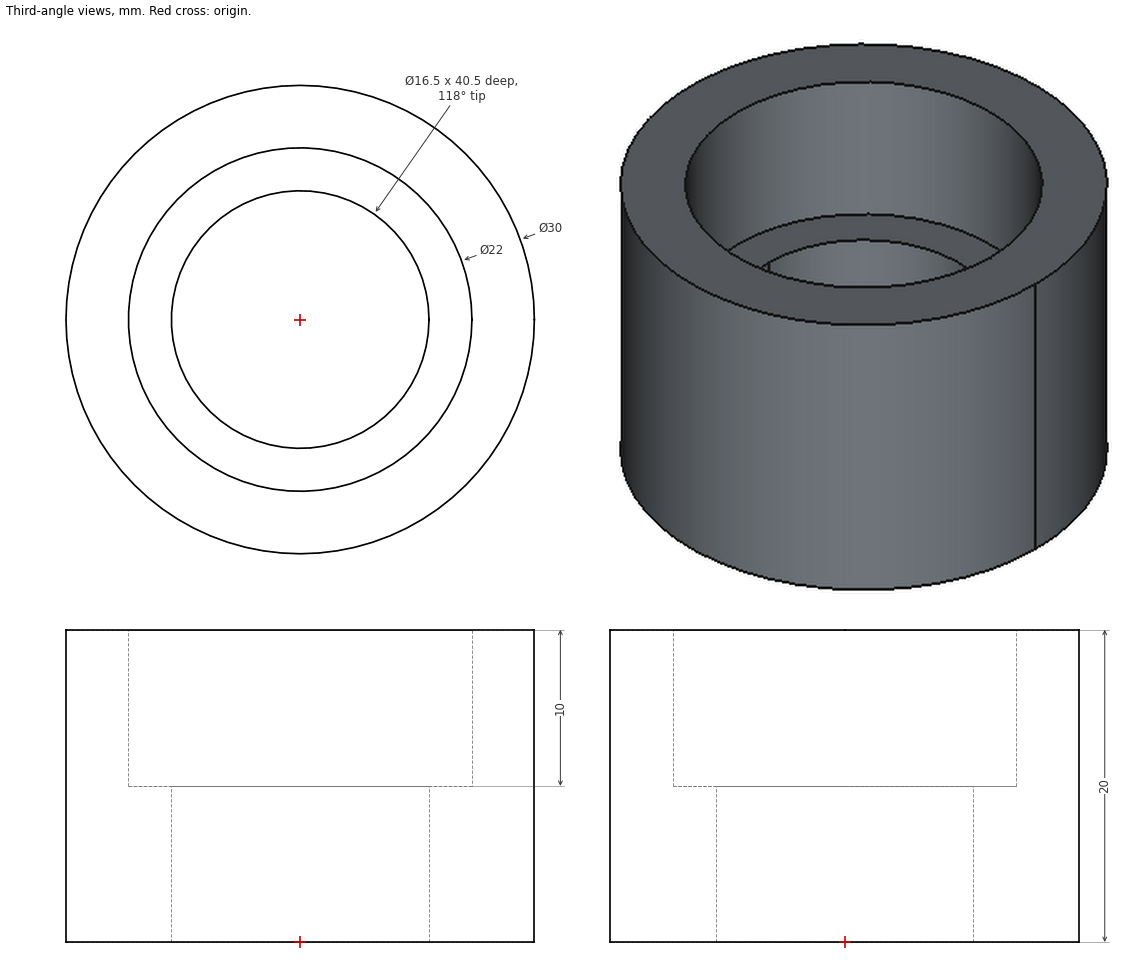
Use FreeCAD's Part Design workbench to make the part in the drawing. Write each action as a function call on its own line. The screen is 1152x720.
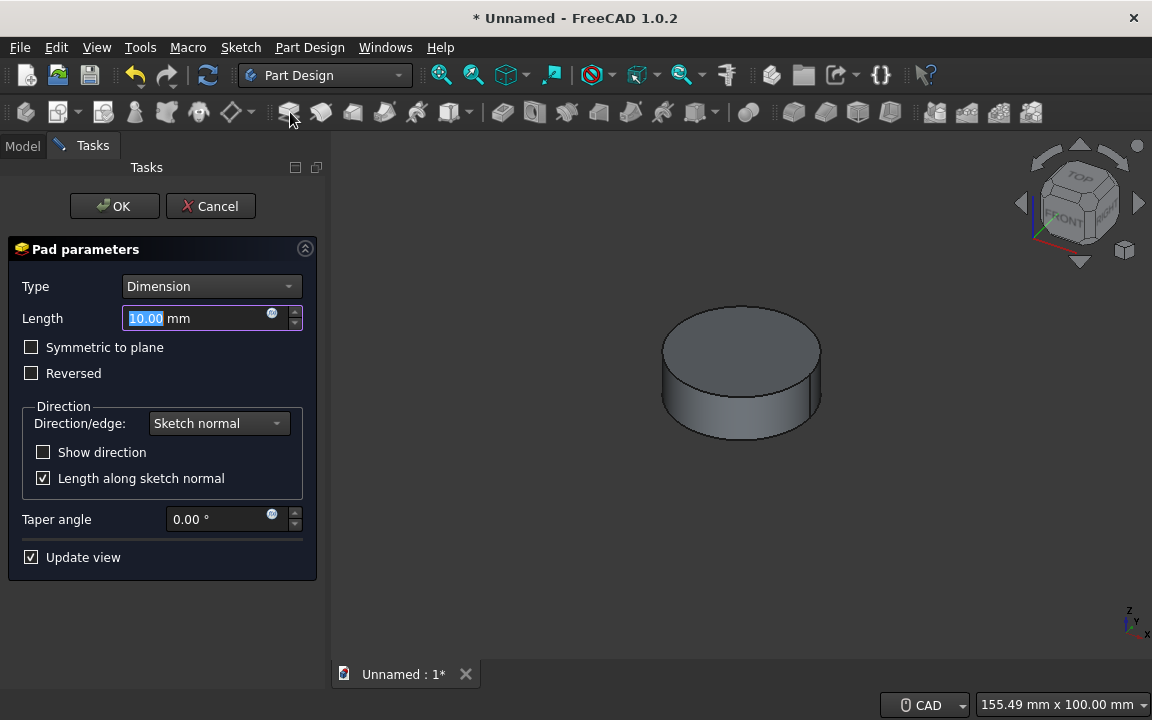
text(20)
key(Tab)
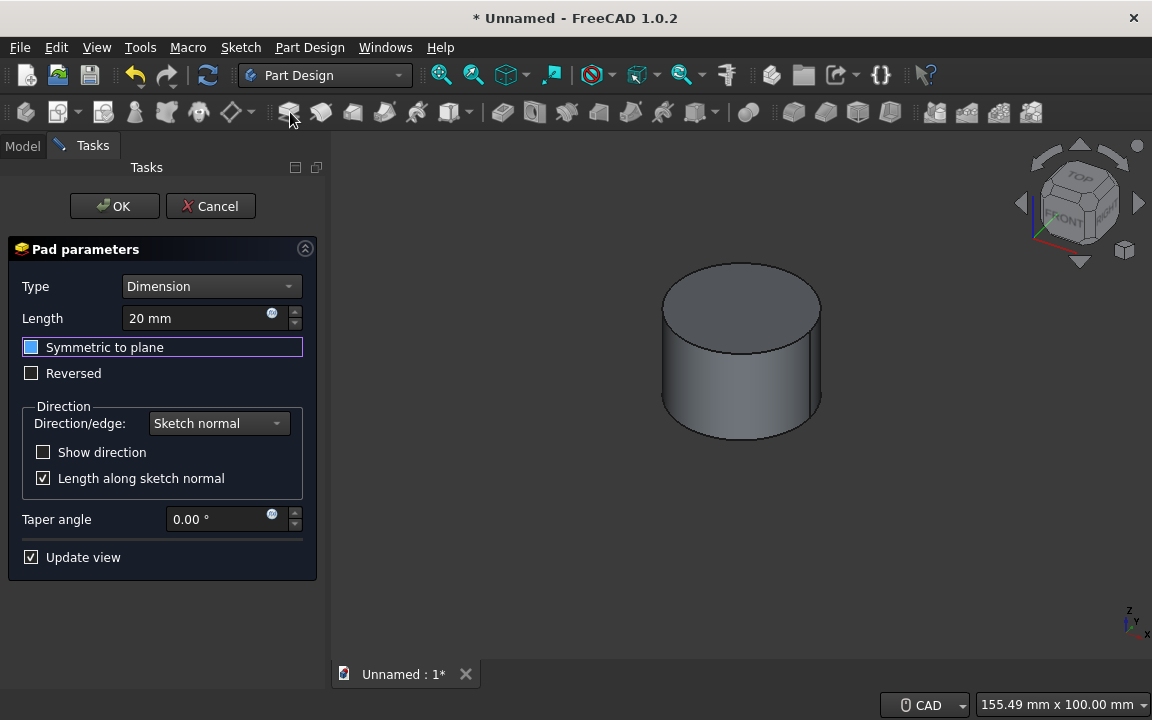
click(115, 206)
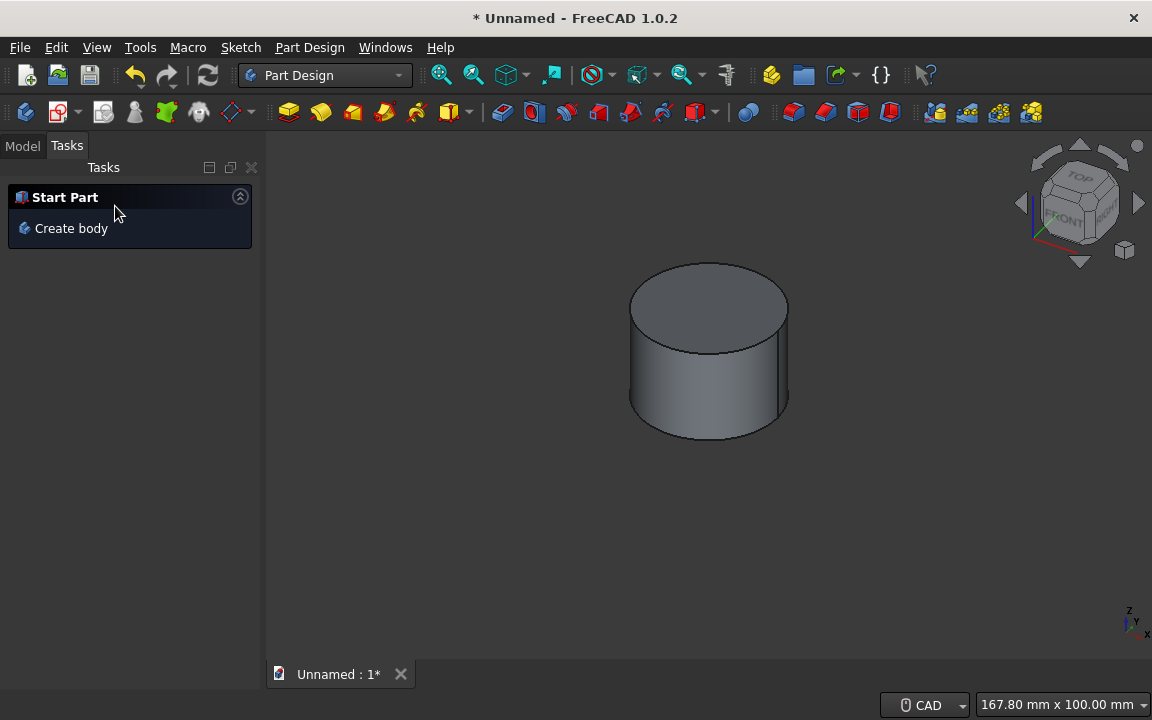
click(442, 76)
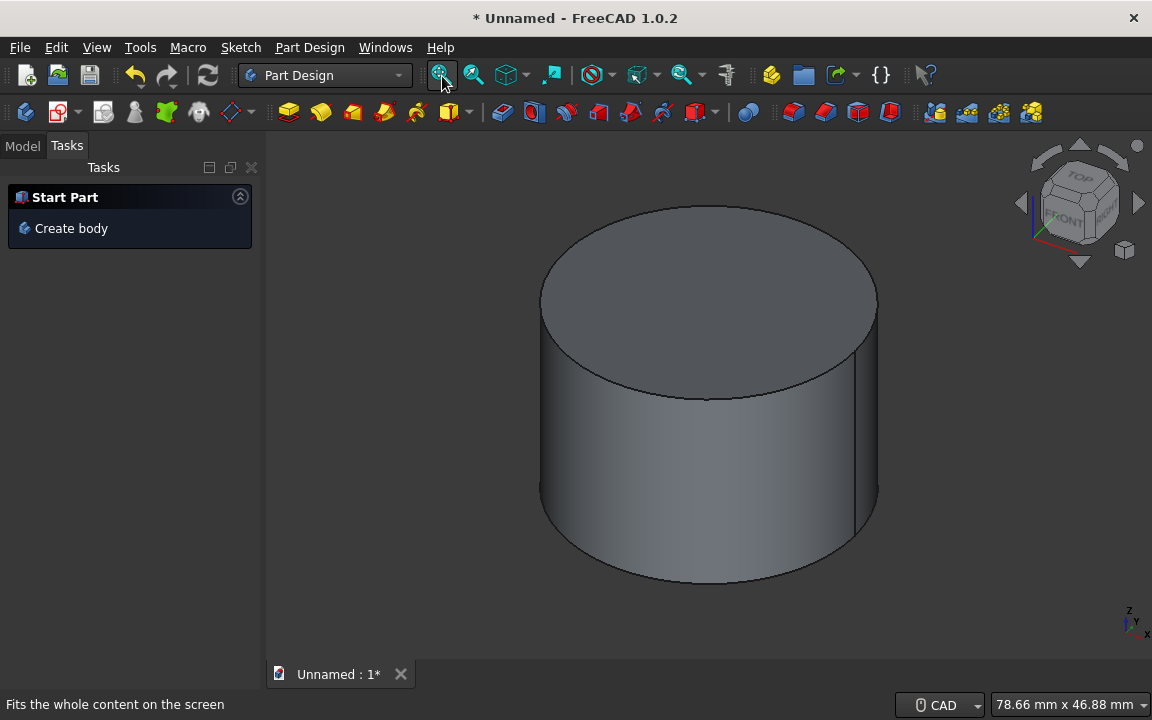
click(709, 302)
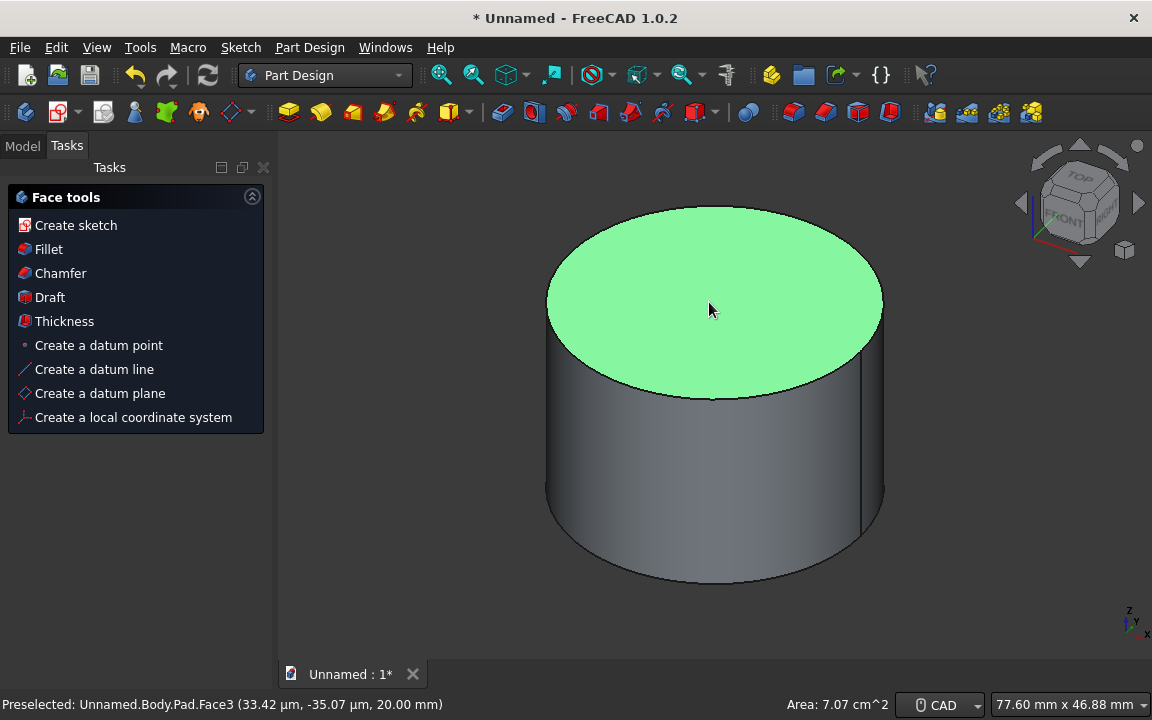
click(58, 112)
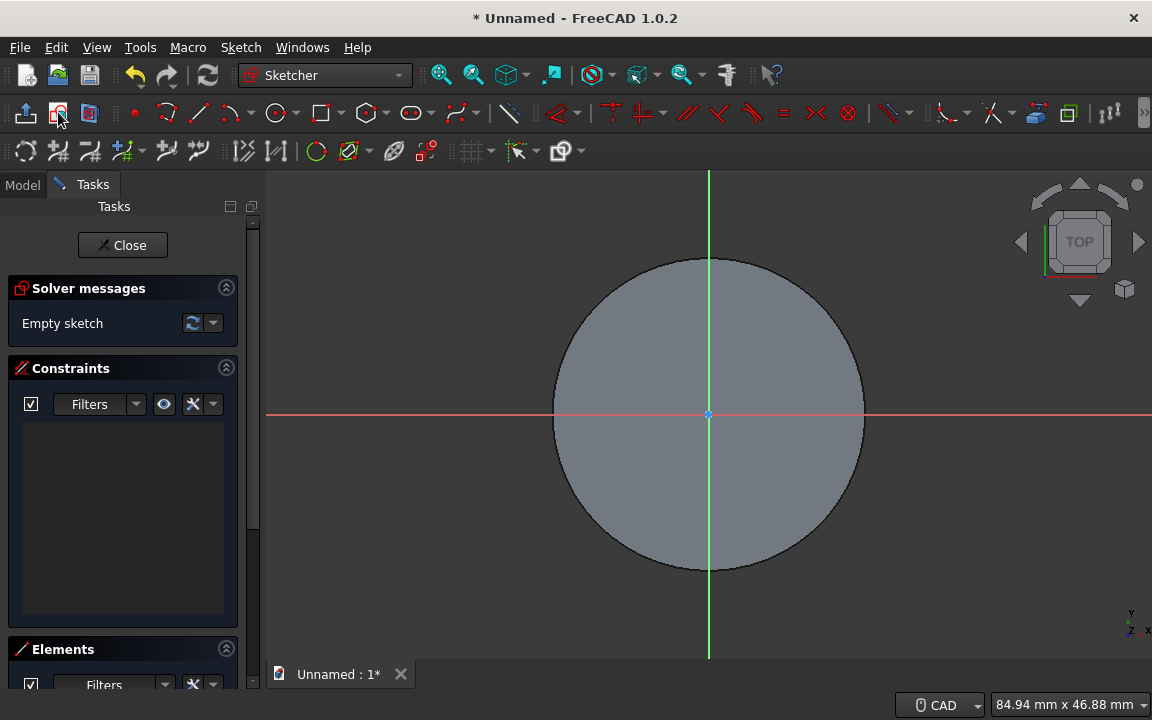
click(276, 114)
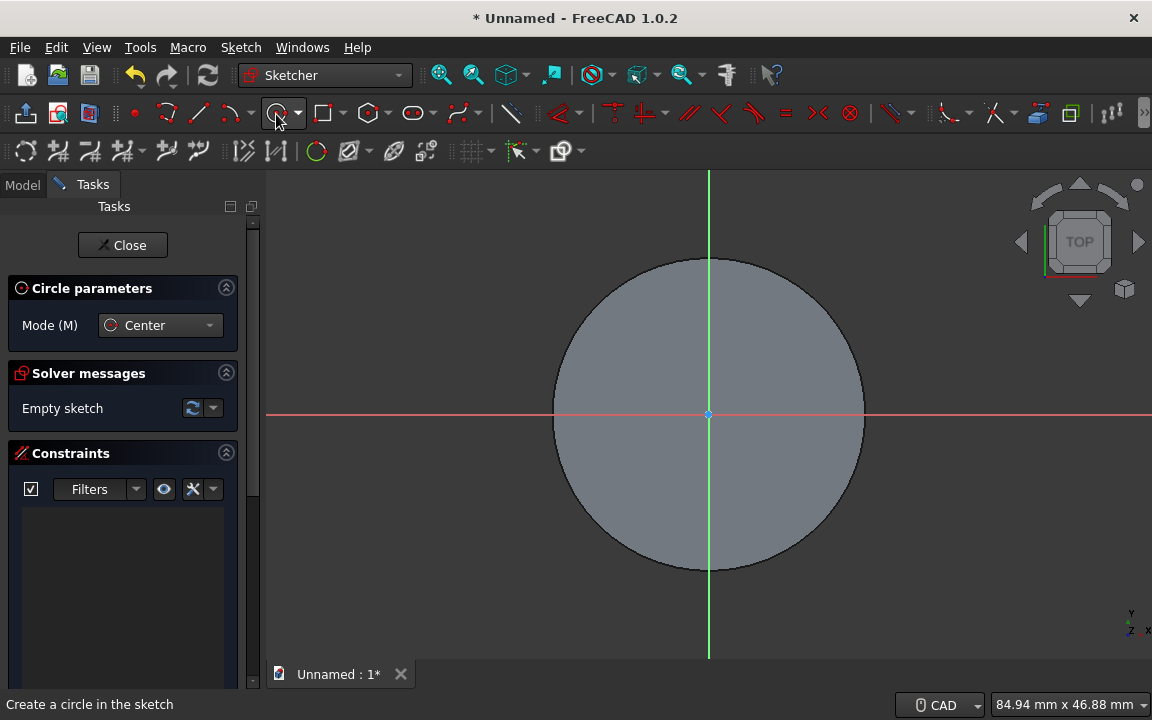
click(709, 414)
click(790, 333)
key(Escape)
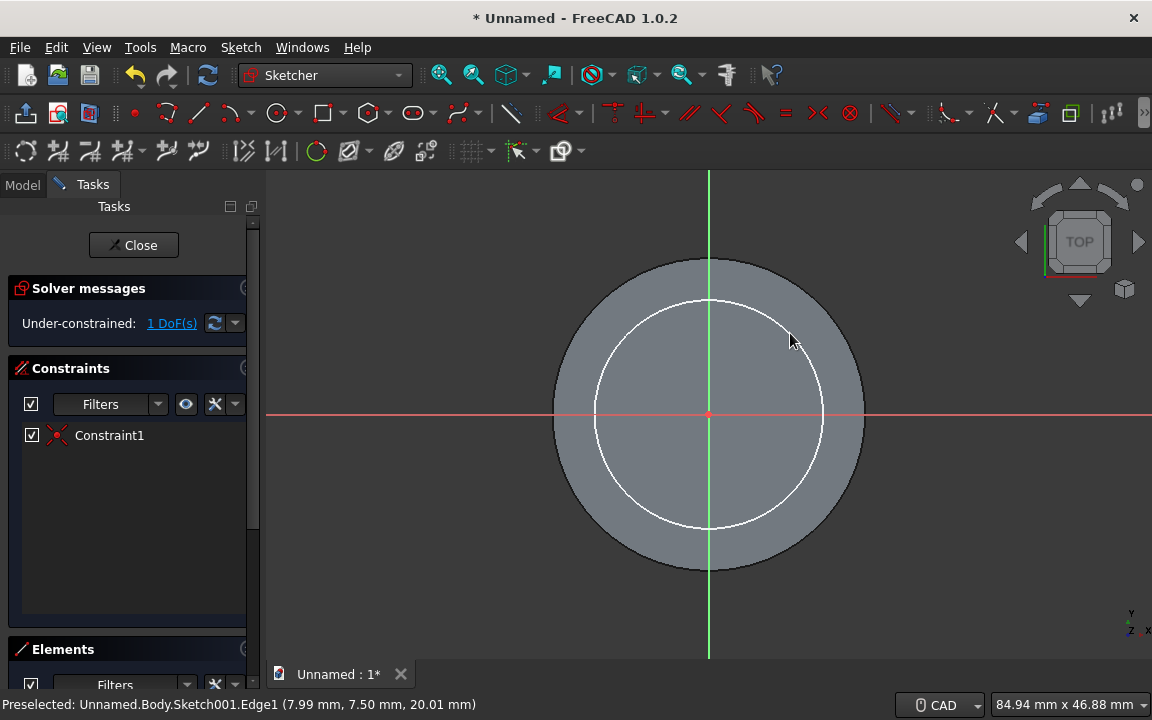
click(558, 114)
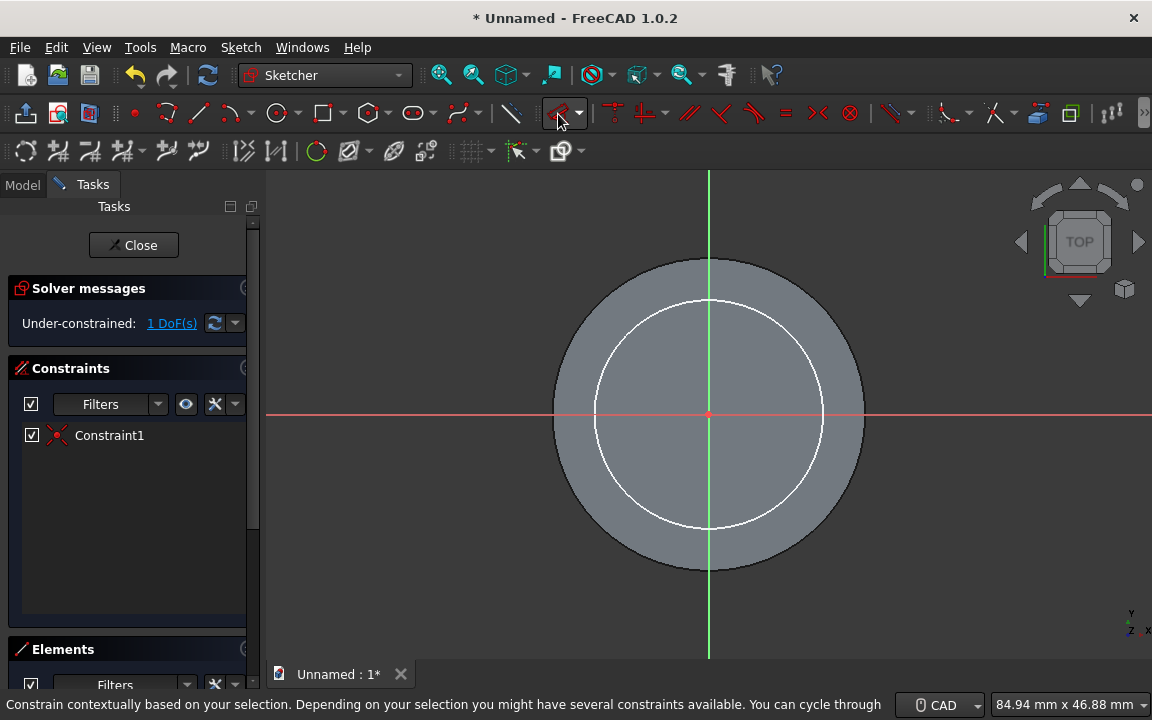
click(789, 333)
click(811, 310)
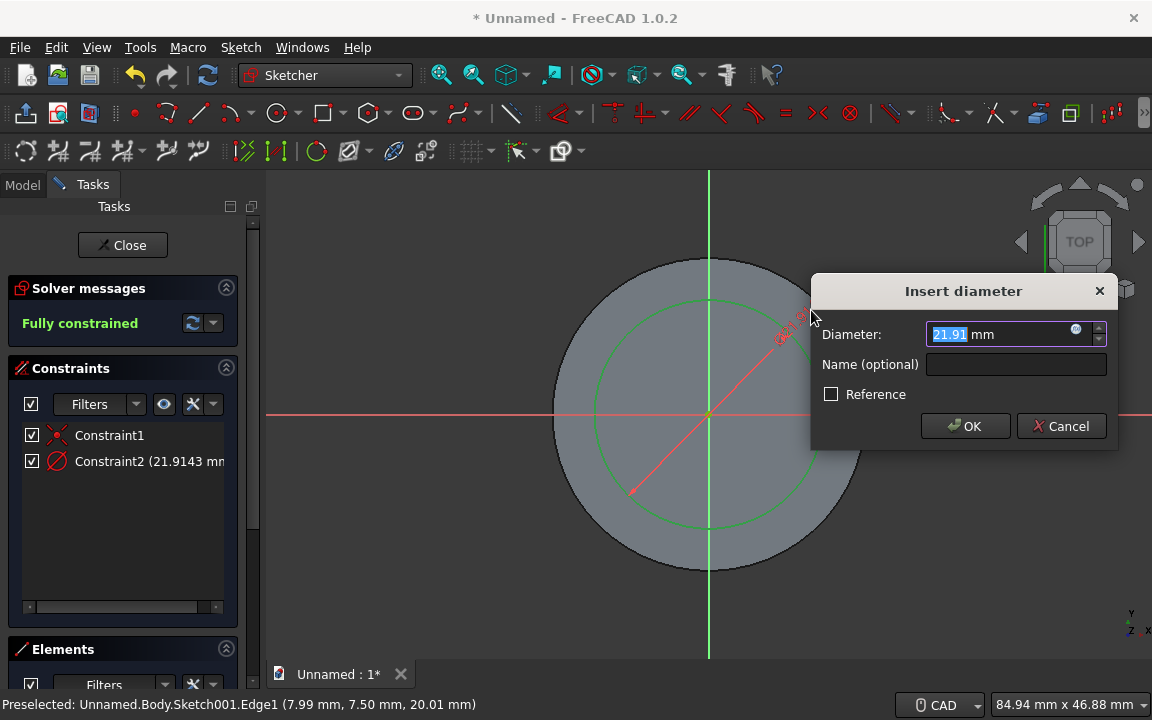
text(22)
key(Return)
key(Escape)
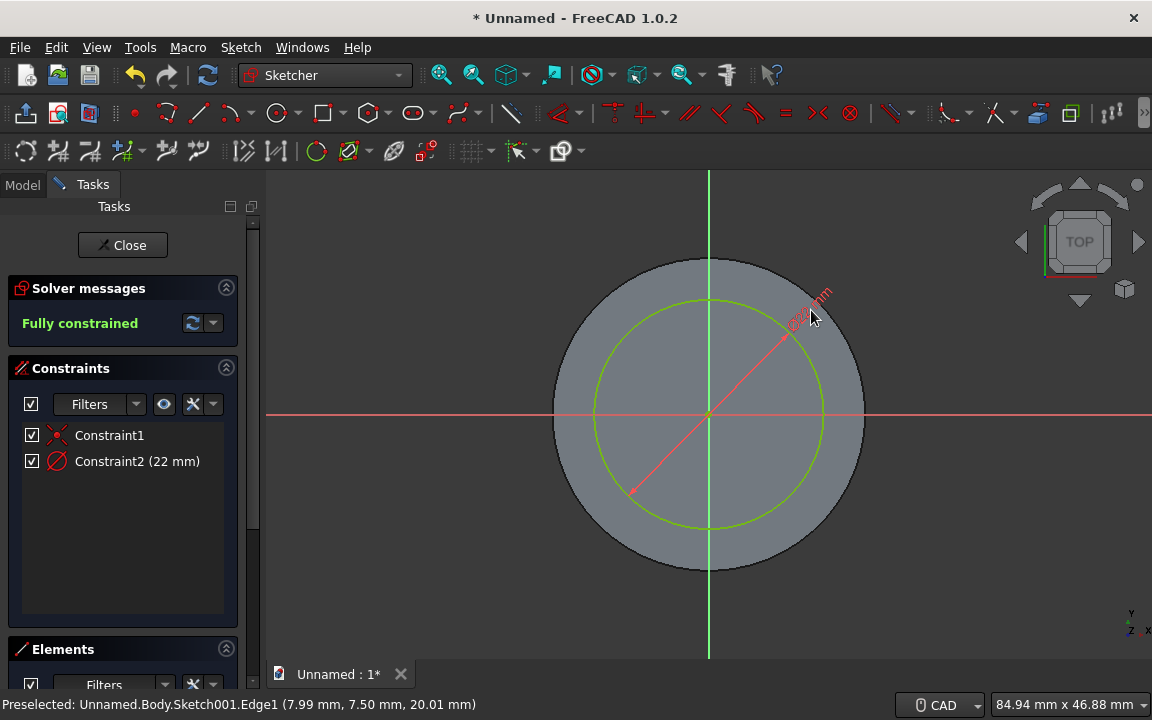
click(123, 245)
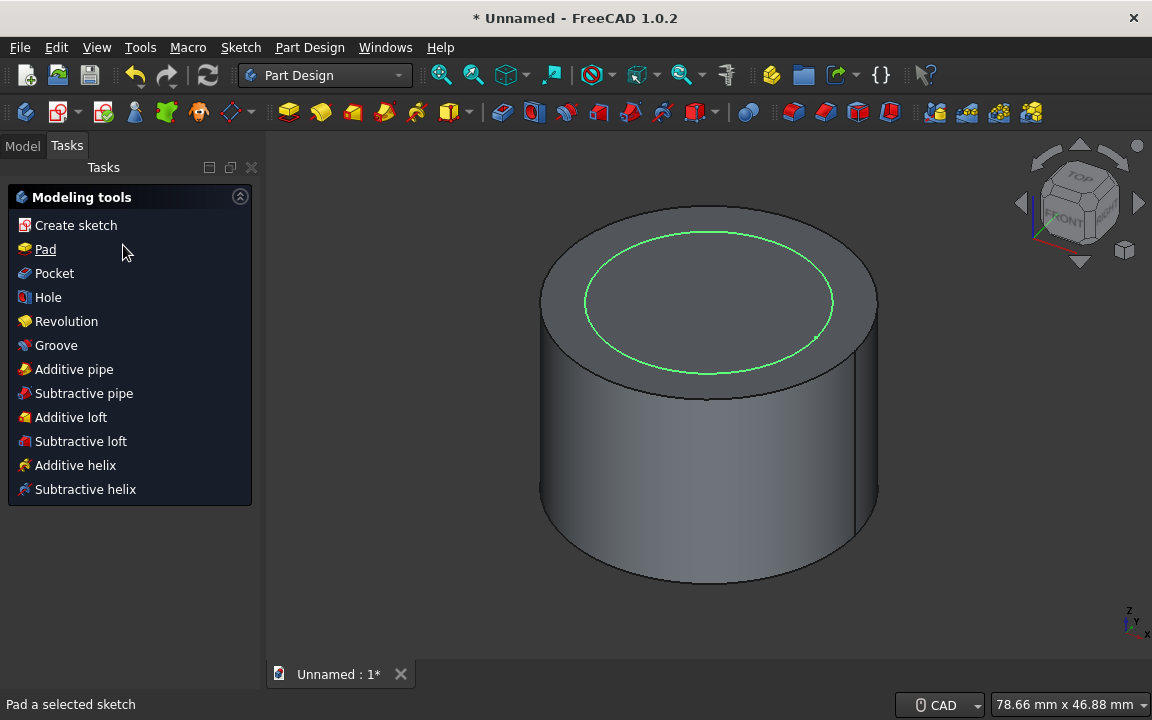
click(504, 112)